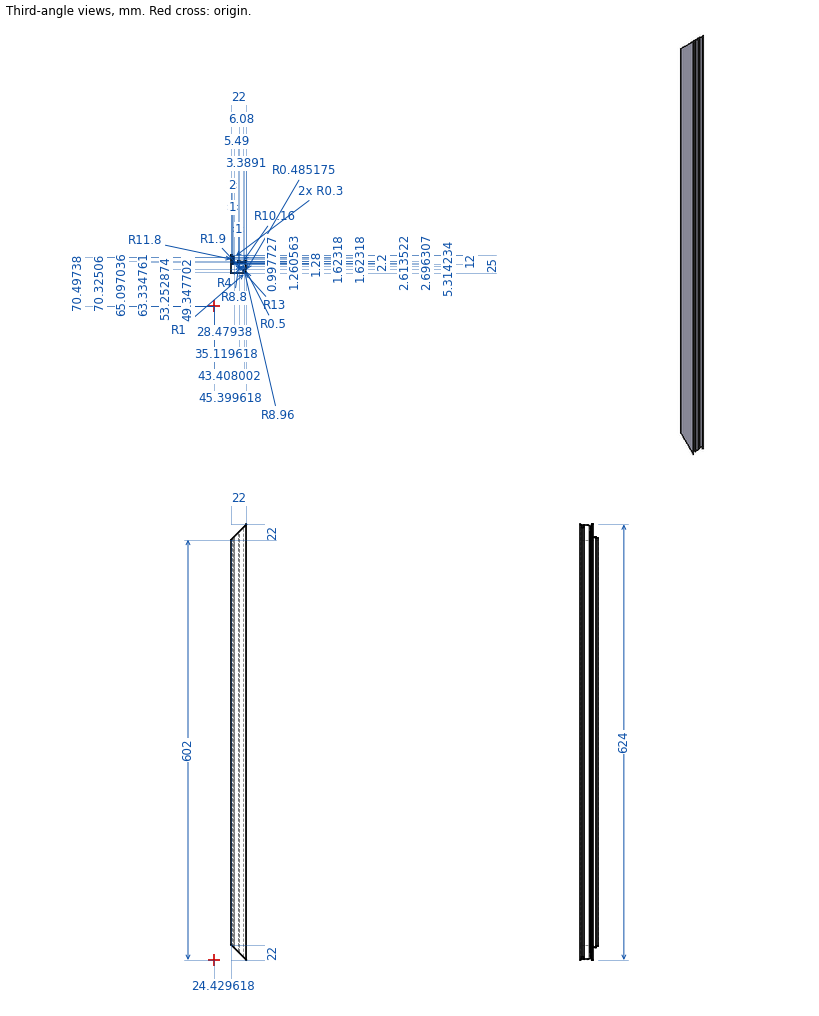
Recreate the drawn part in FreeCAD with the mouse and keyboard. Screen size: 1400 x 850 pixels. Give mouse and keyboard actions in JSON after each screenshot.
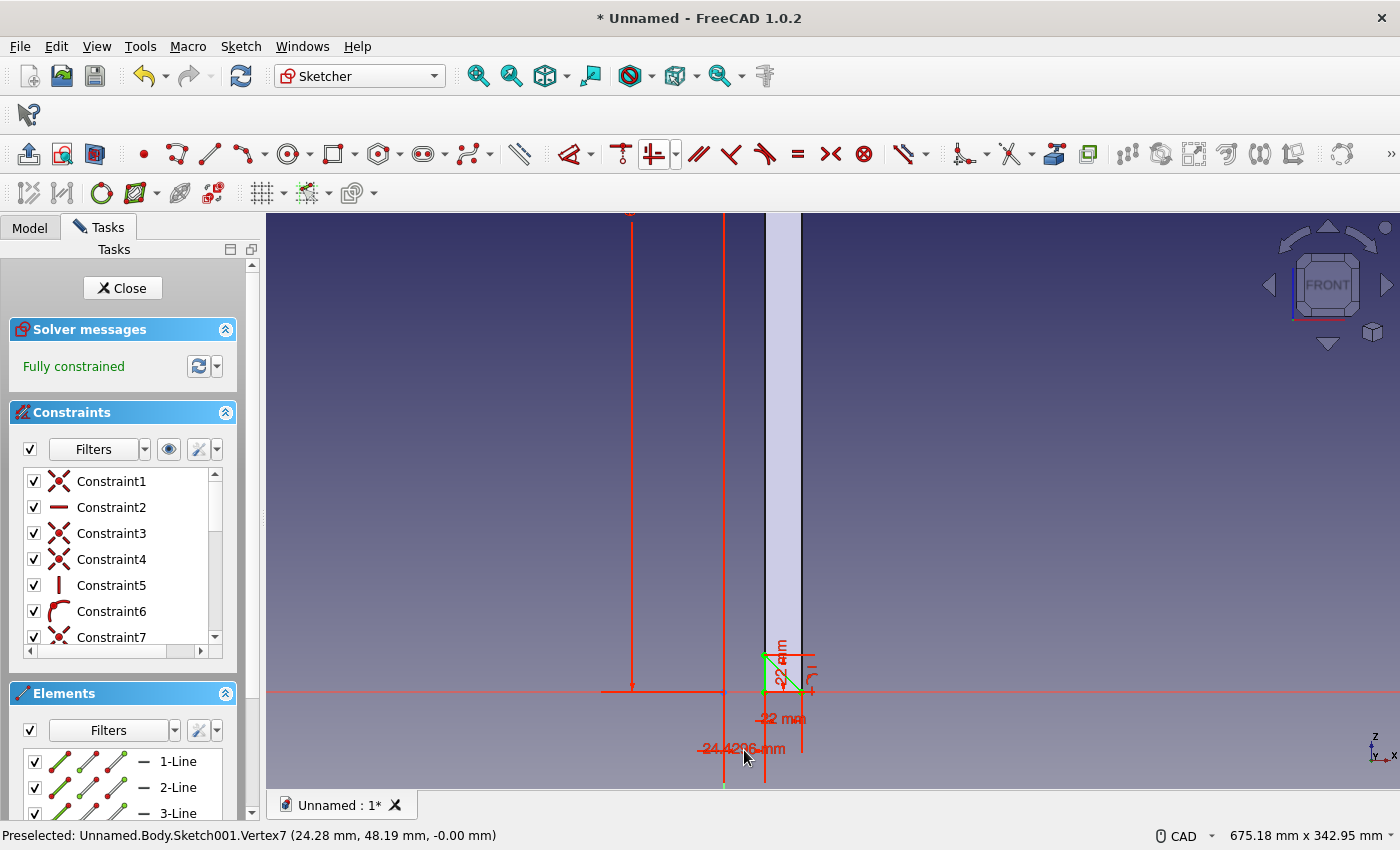
{"action": "left_click", "coordinate": [123, 288]}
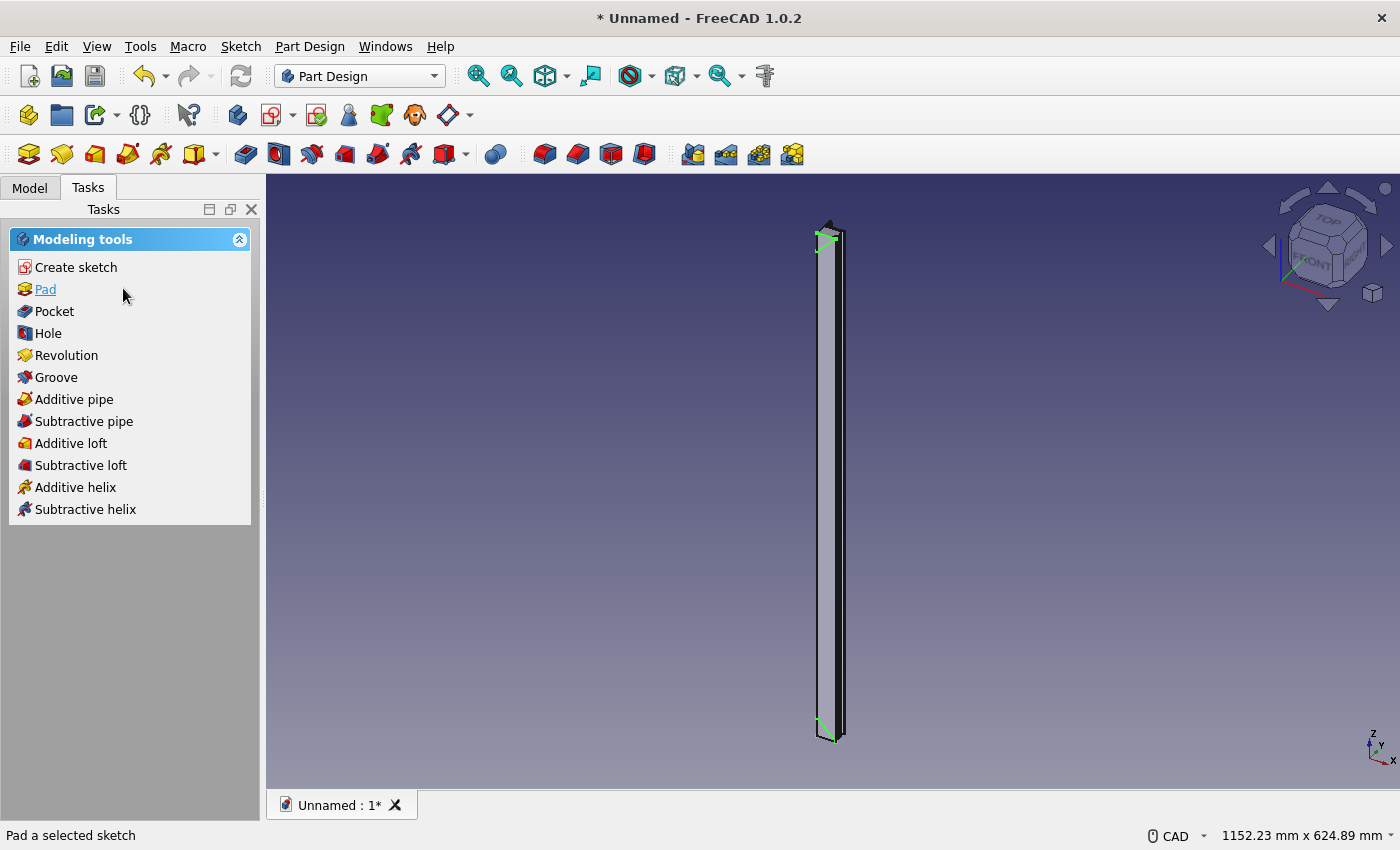
{"action": "left_click", "coordinate": [246, 154]}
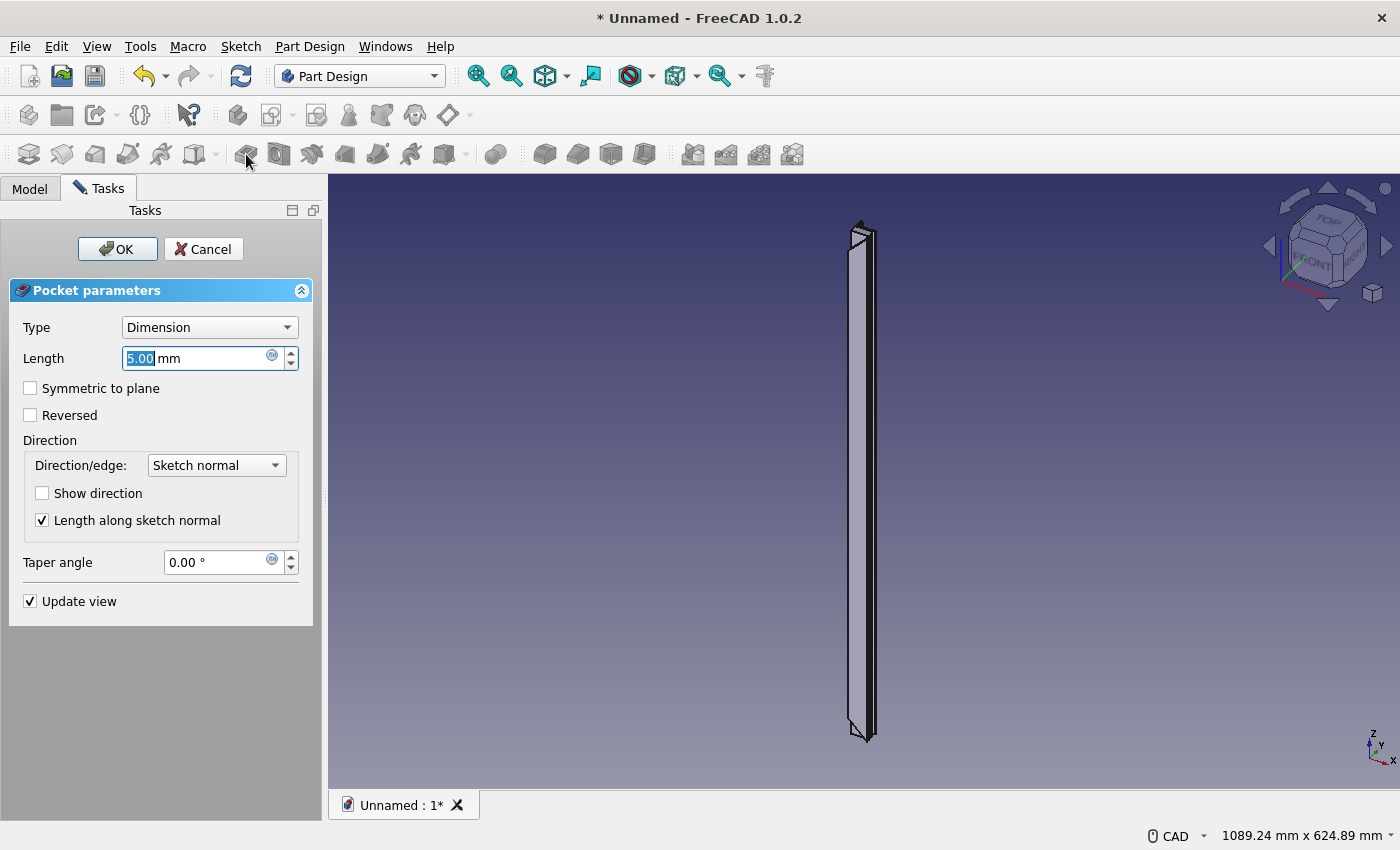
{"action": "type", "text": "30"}
{"action": "key", "text": "Tab"}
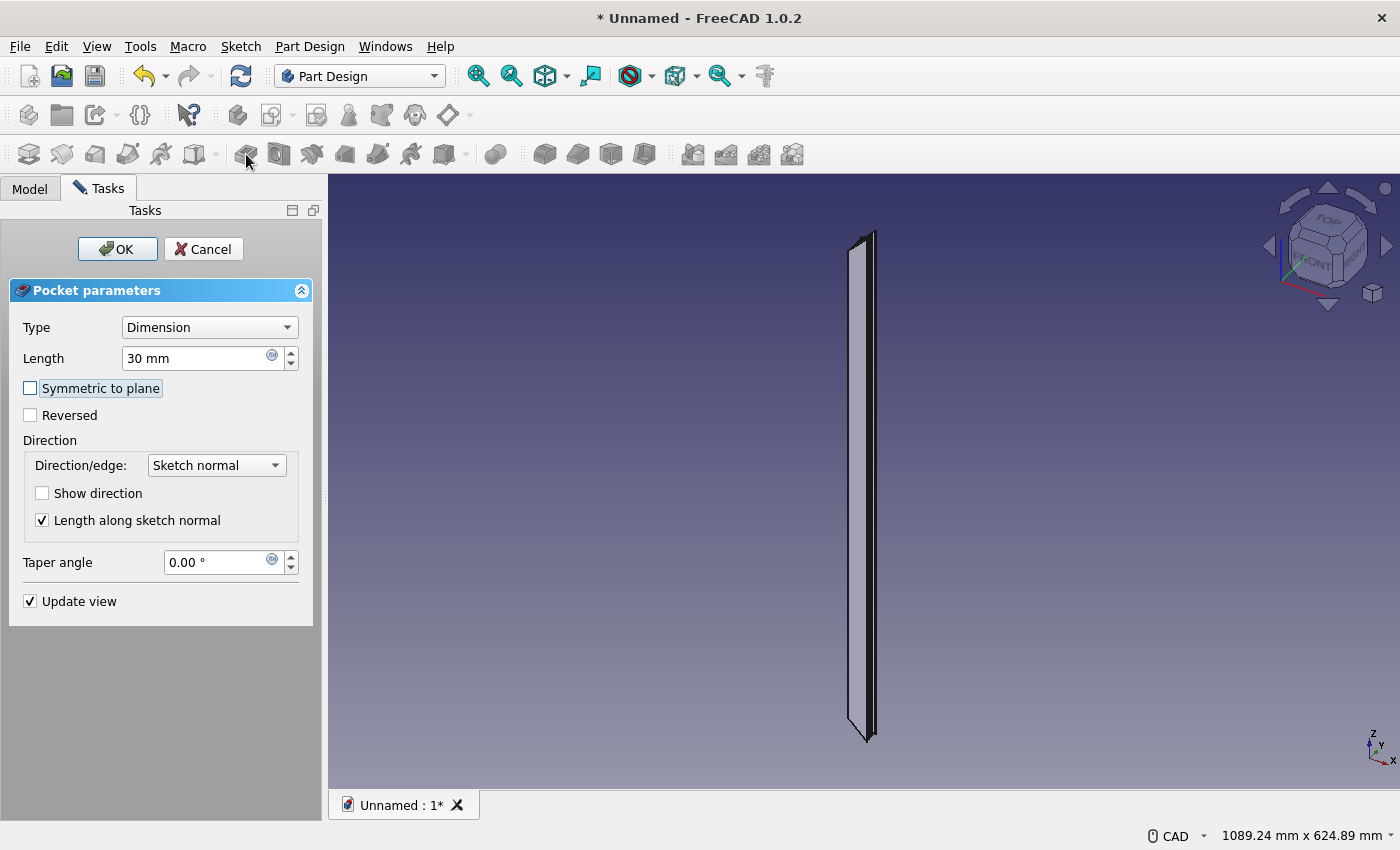
{"action": "left_click", "coordinate": [118, 249]}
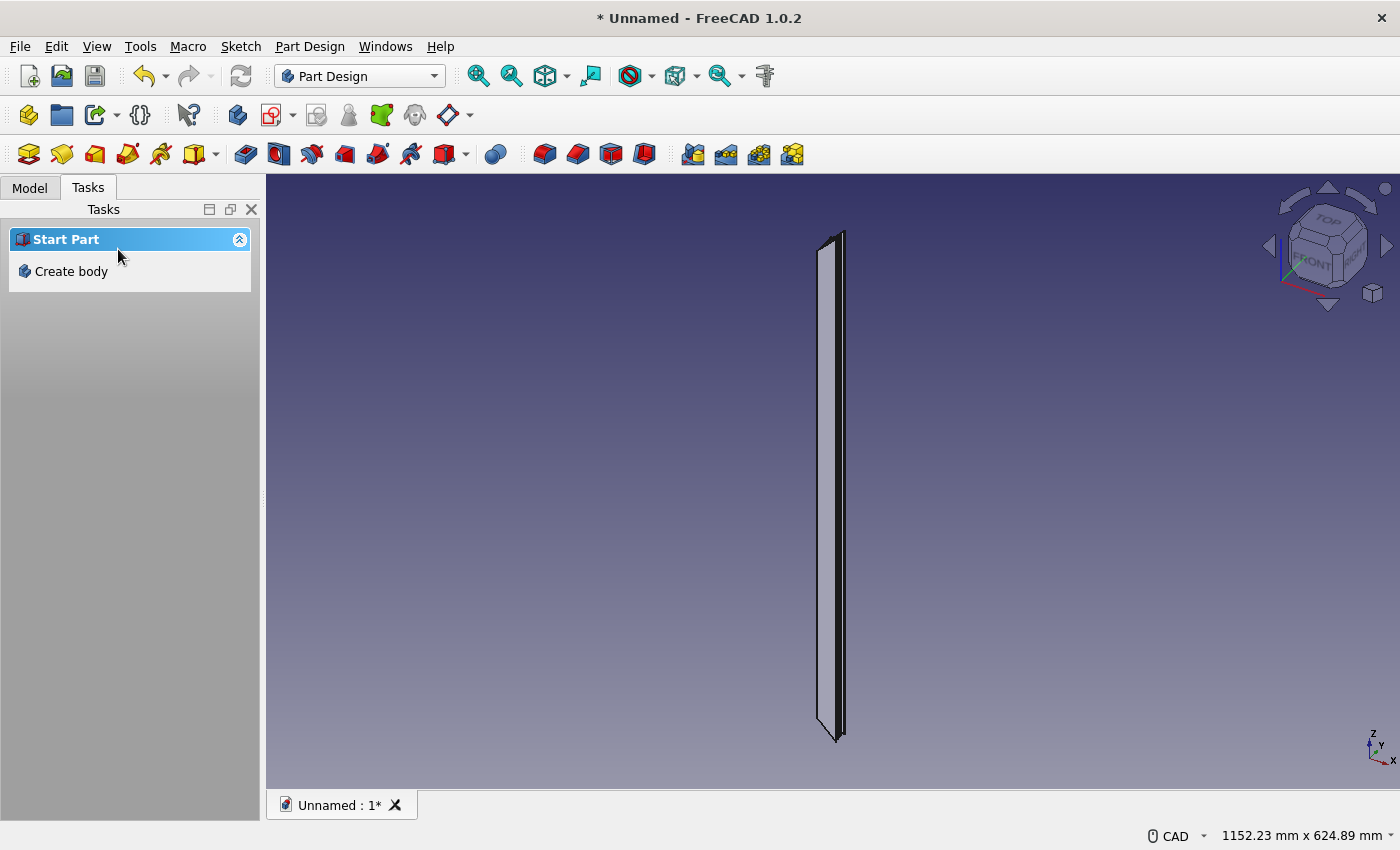
{"action": "key", "text": "0"}